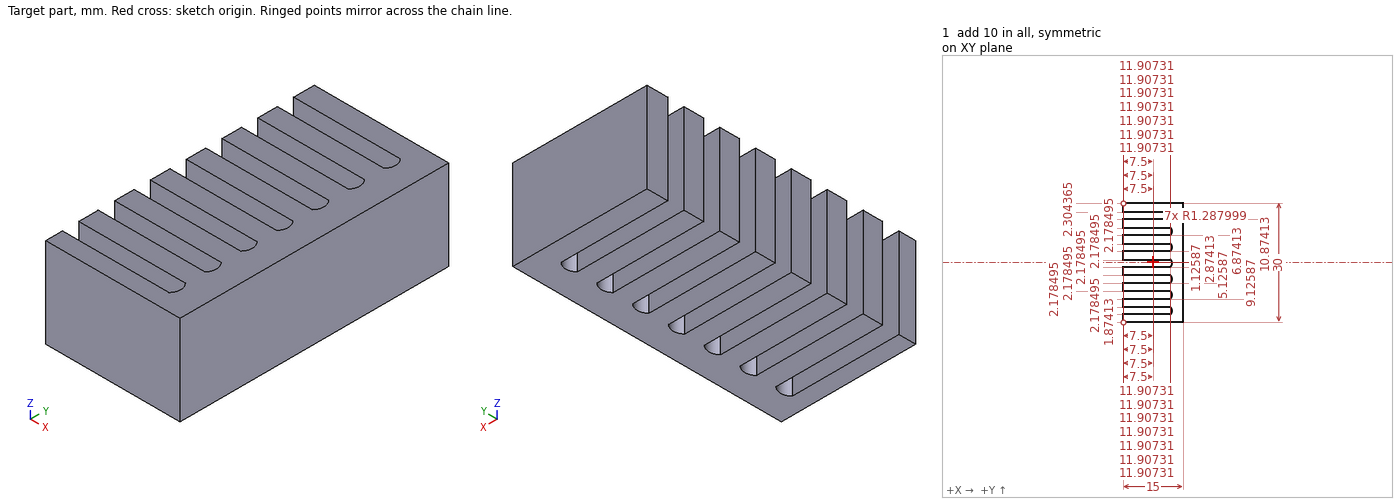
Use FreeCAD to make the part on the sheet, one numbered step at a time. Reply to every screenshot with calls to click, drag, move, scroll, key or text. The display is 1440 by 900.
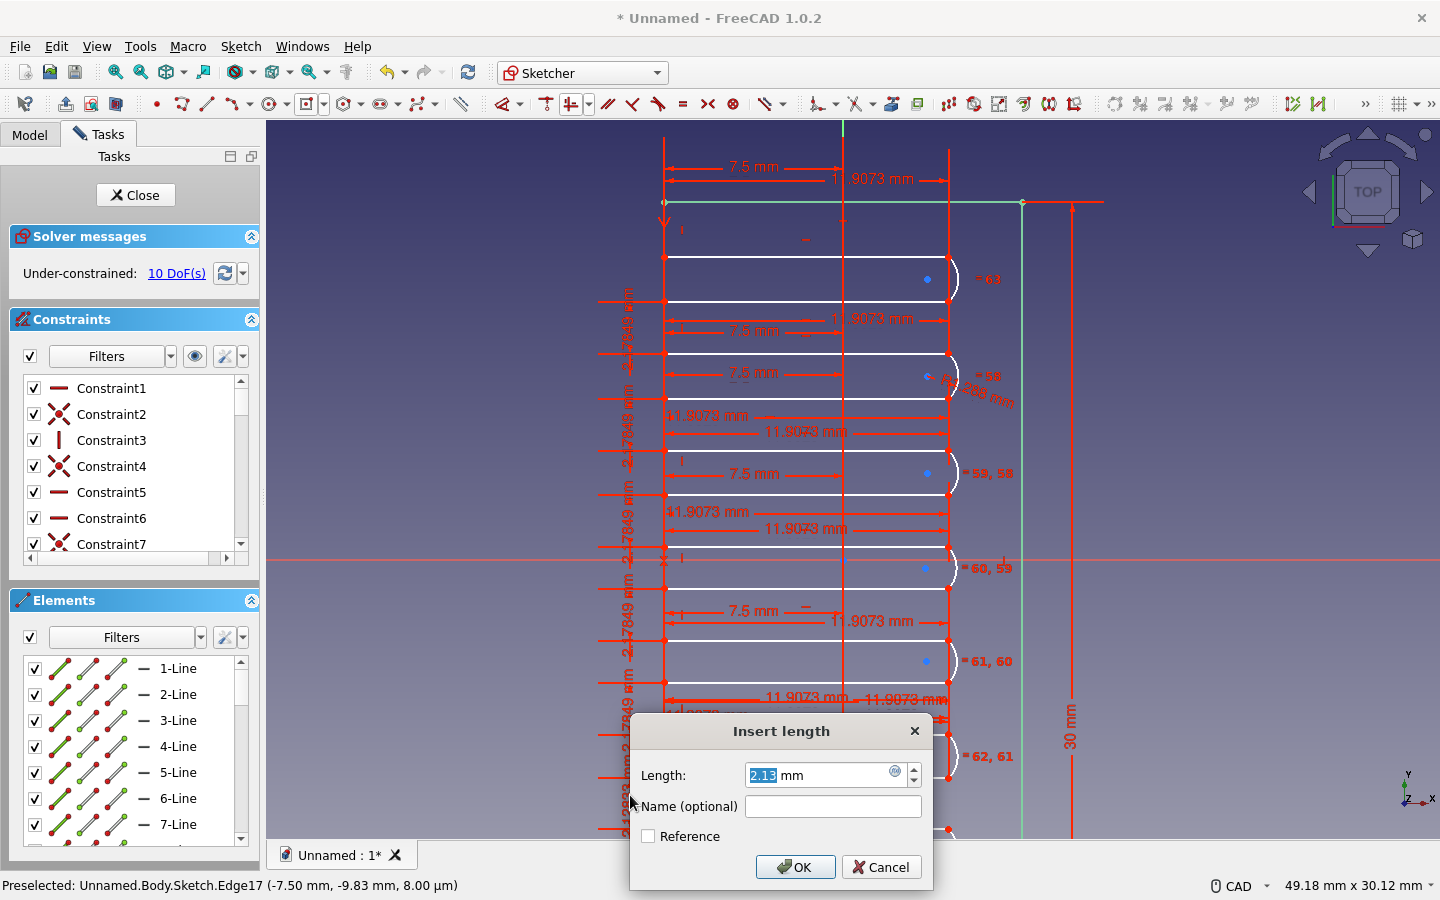
text(2.178495)
key(Return)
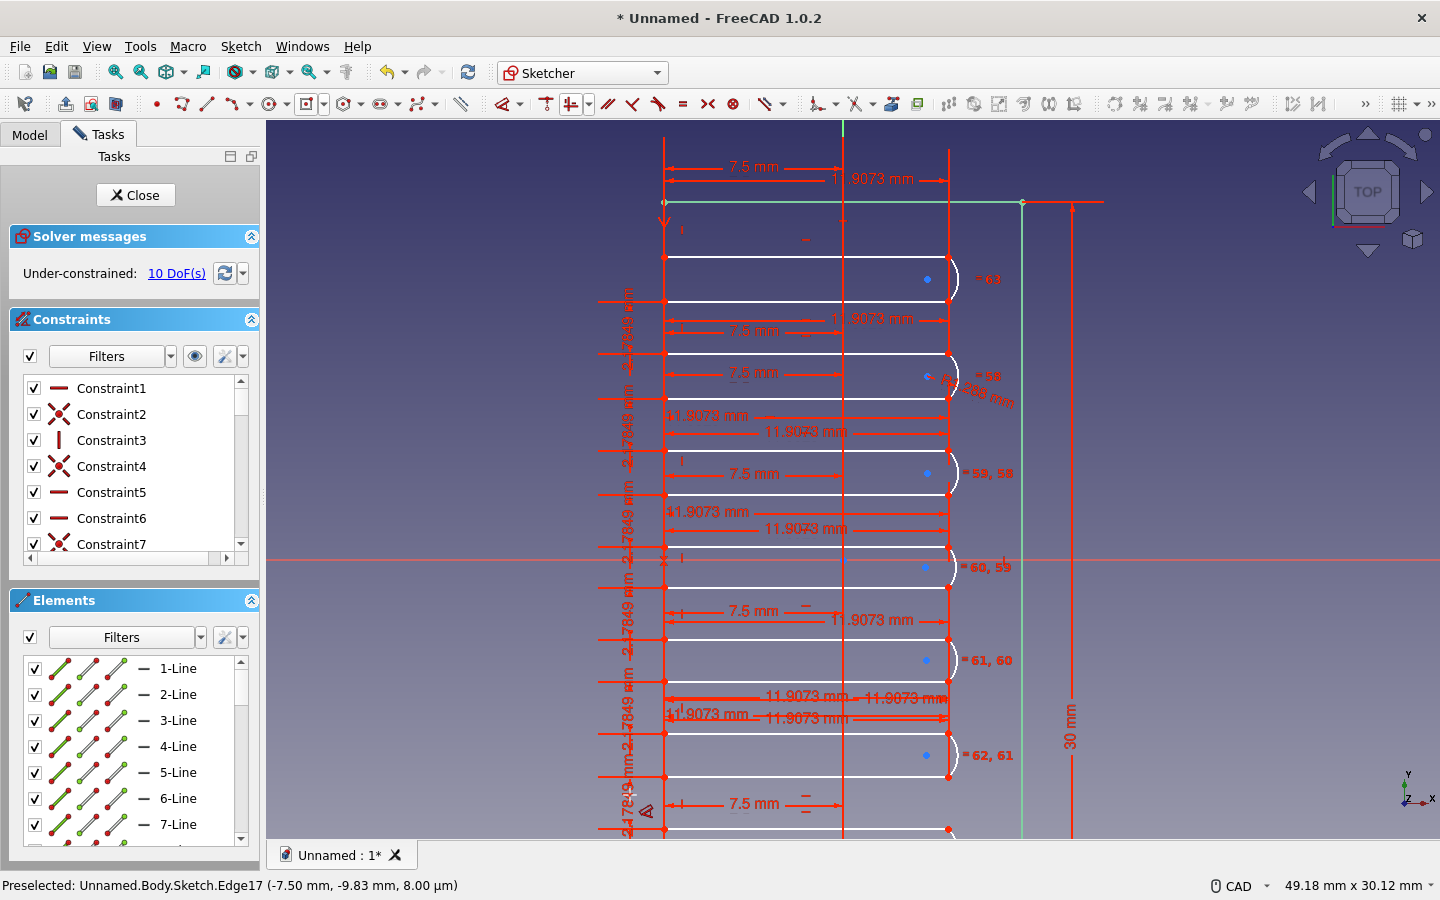
scroll(665, 315, down, 2)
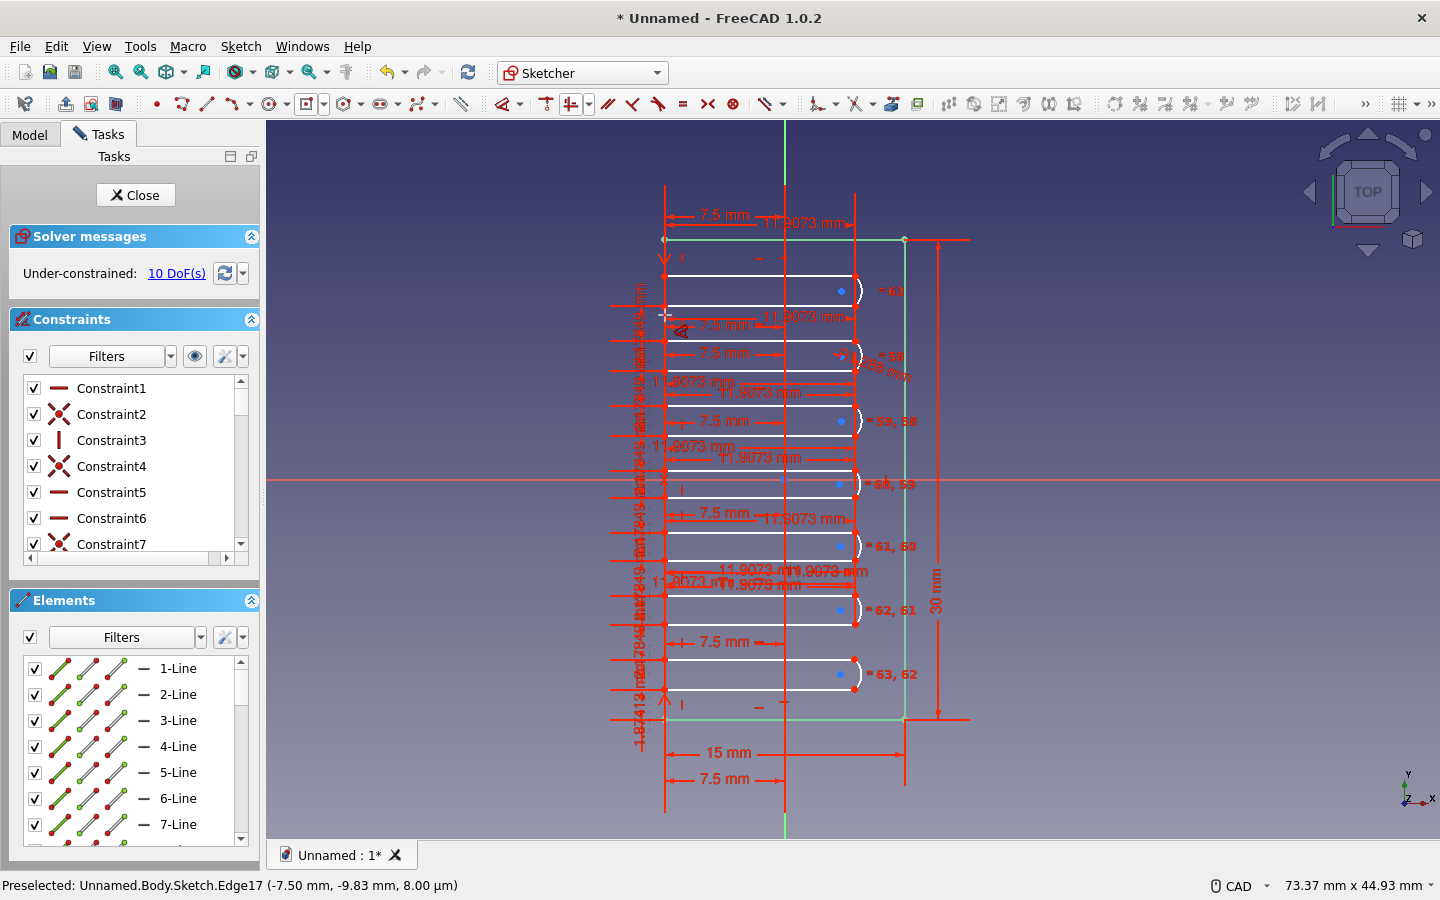
click(722, 660)
click(804, 742)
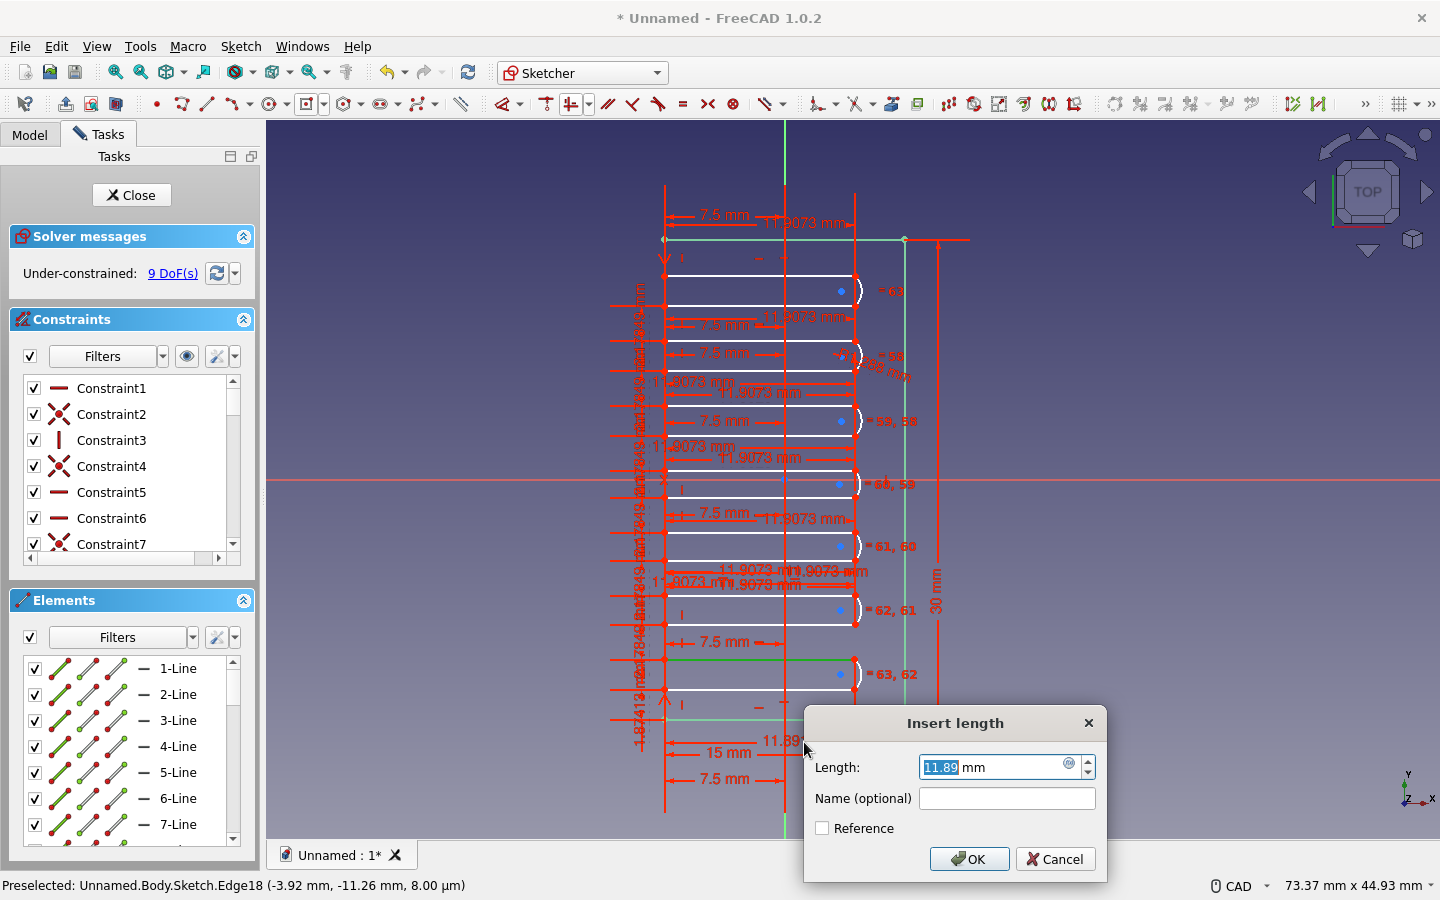
text(11.90731)
key(Return)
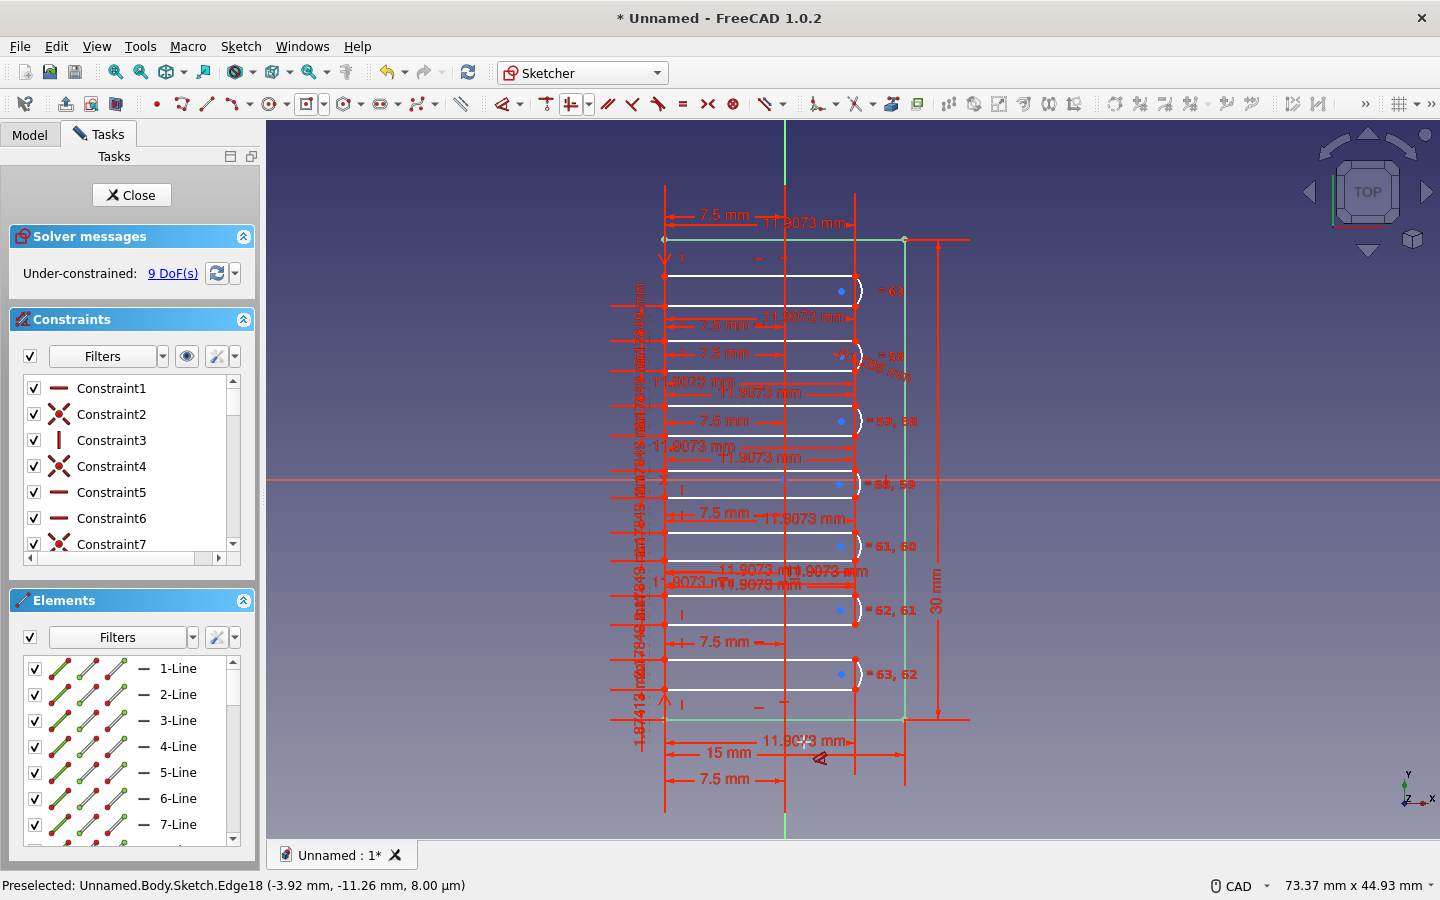
click(798, 690)
click(804, 772)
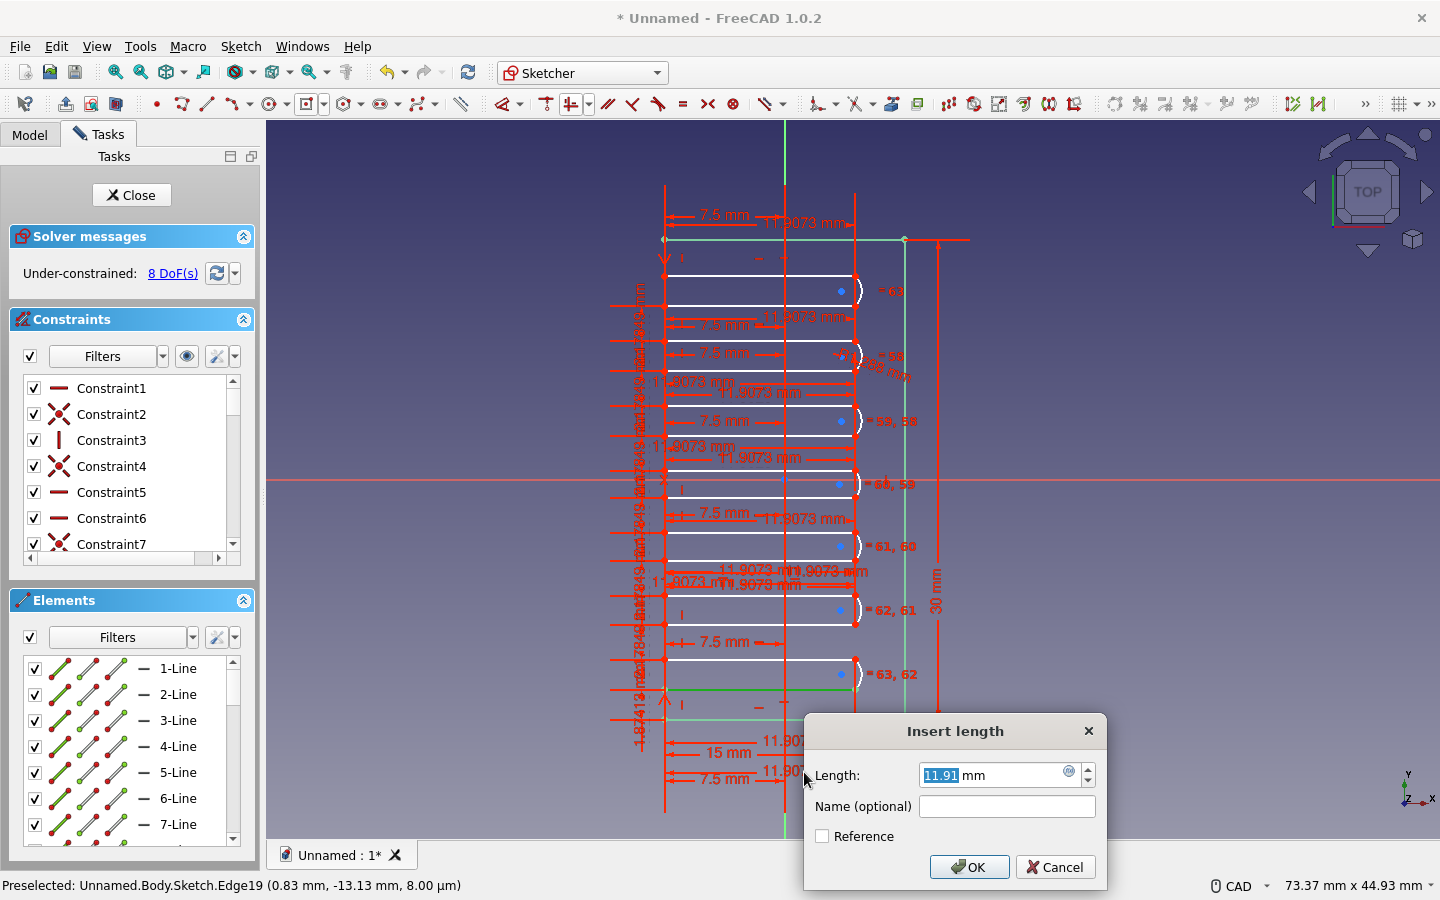
text(11.90731)
key(Return)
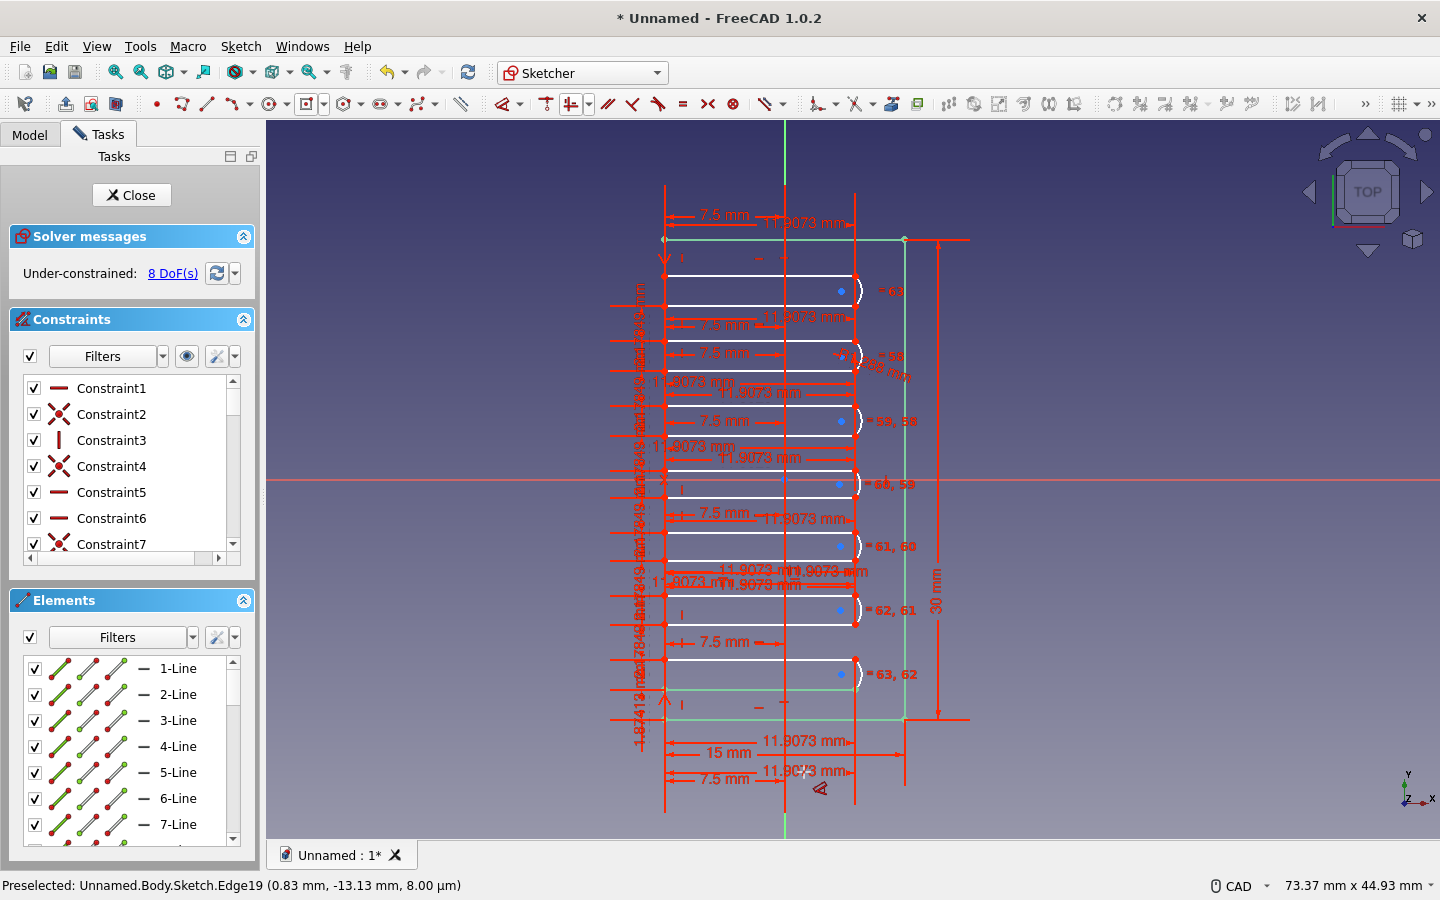
scroll(665, 251, up, 2)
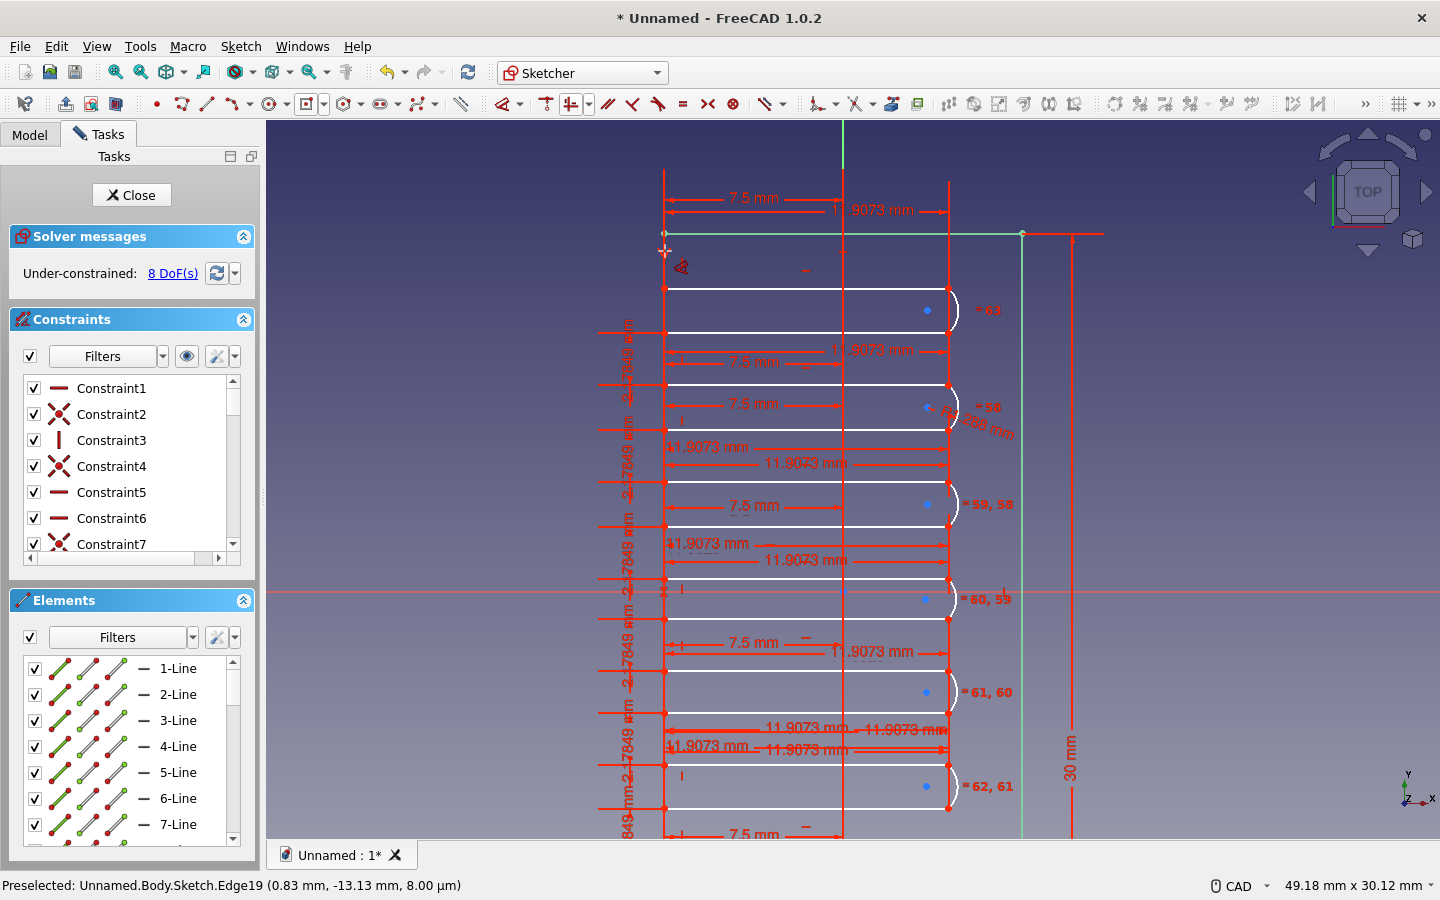
click(664, 250)
click(630, 261)